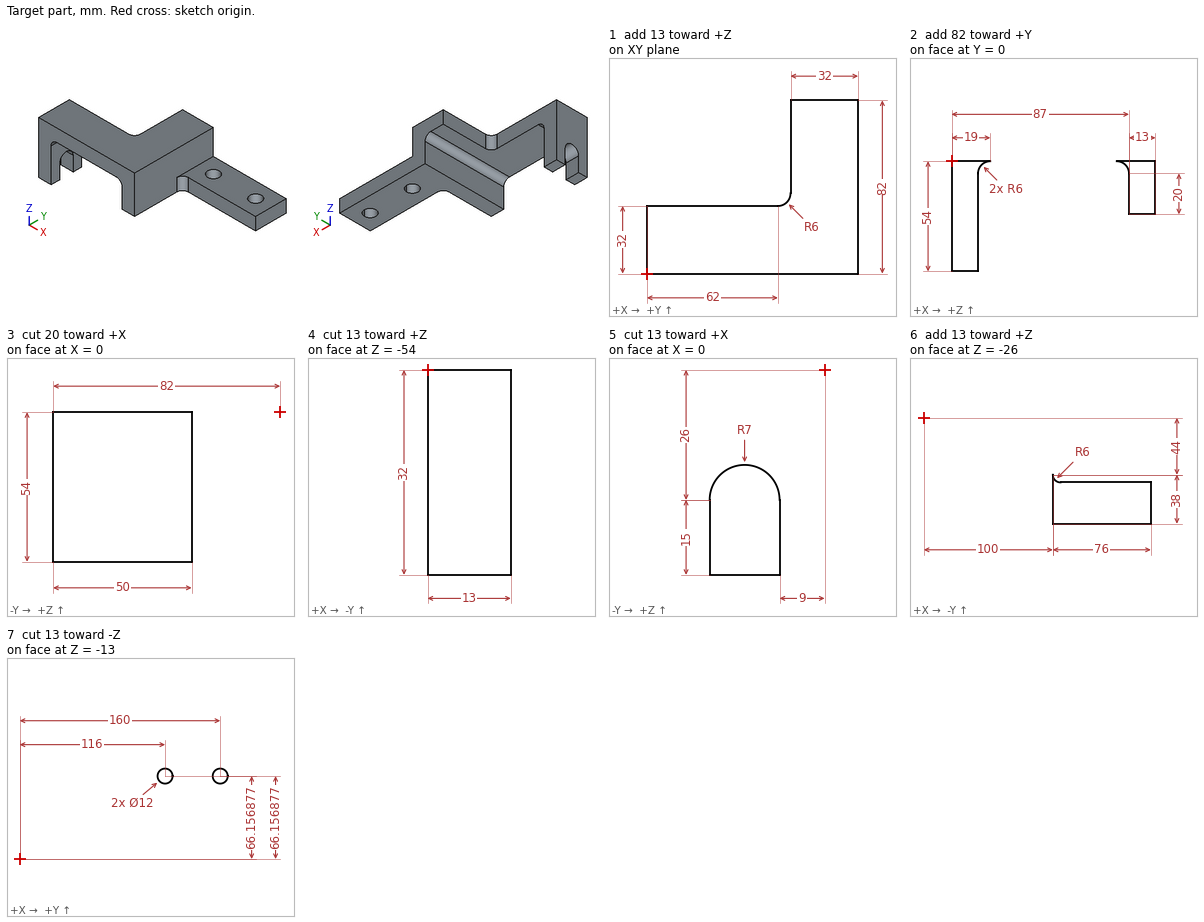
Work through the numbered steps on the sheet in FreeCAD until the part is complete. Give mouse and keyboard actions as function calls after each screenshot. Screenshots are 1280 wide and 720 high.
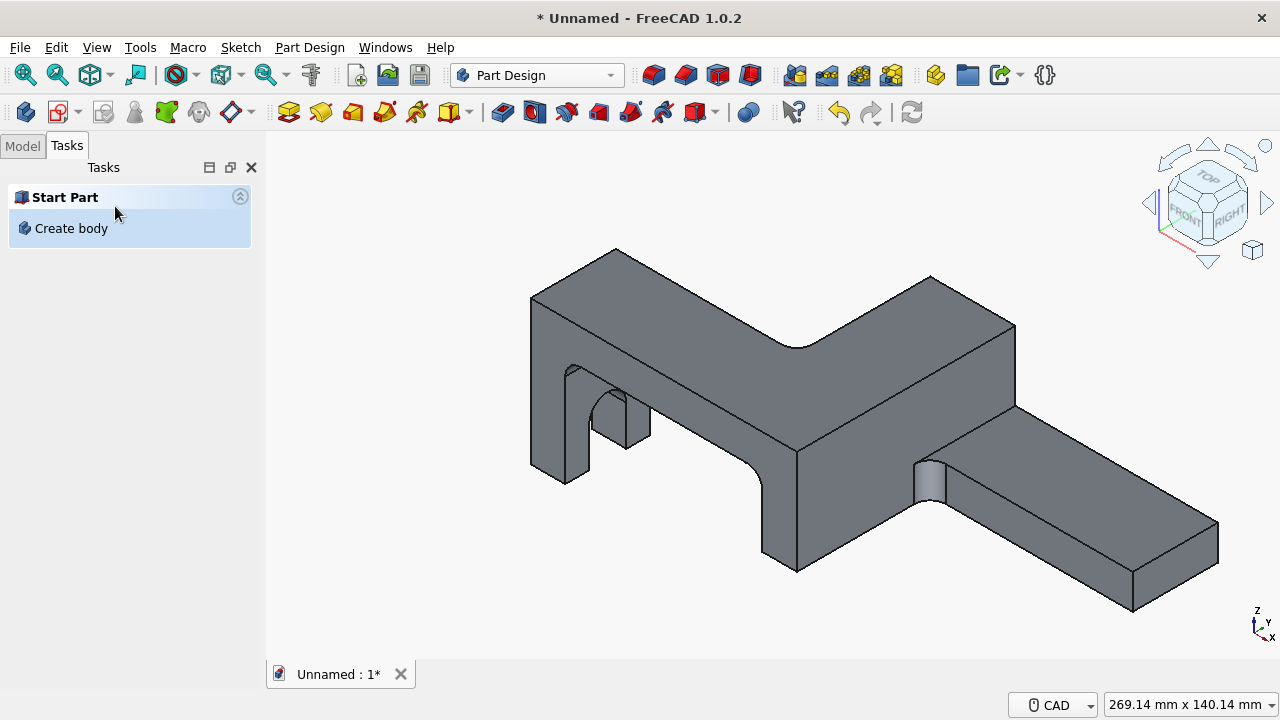
click(26, 76)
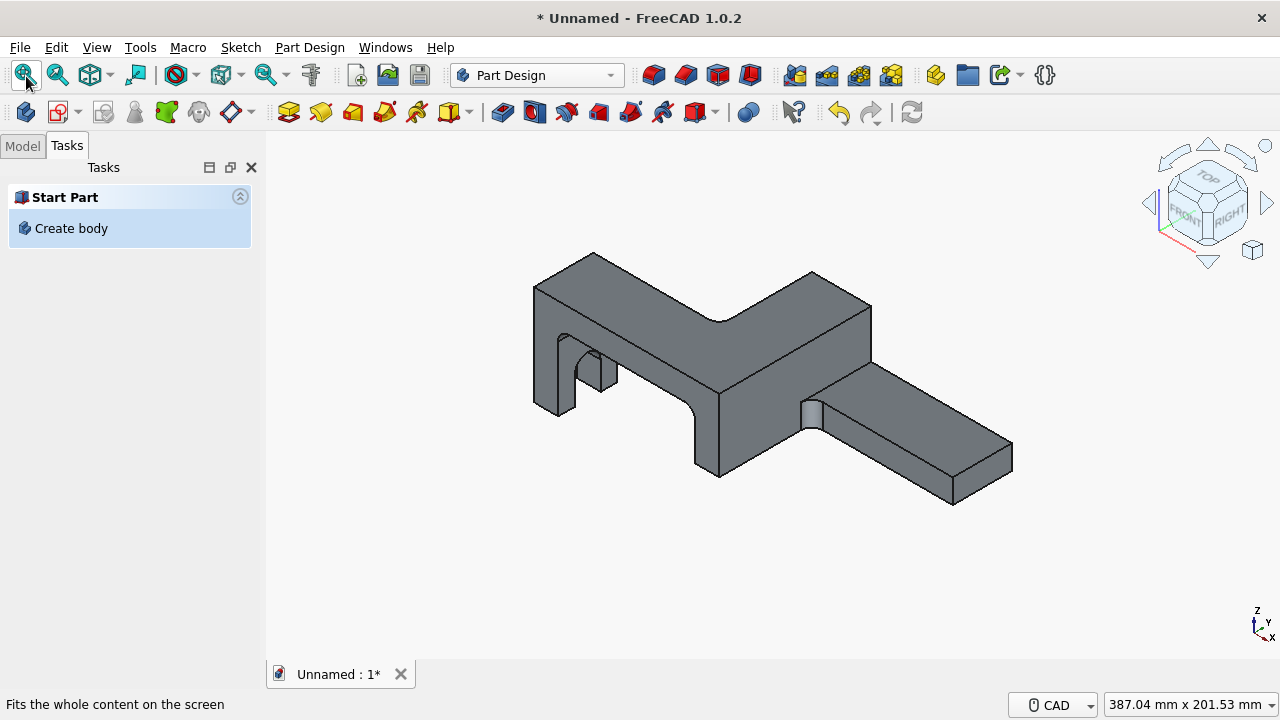
click(957, 439)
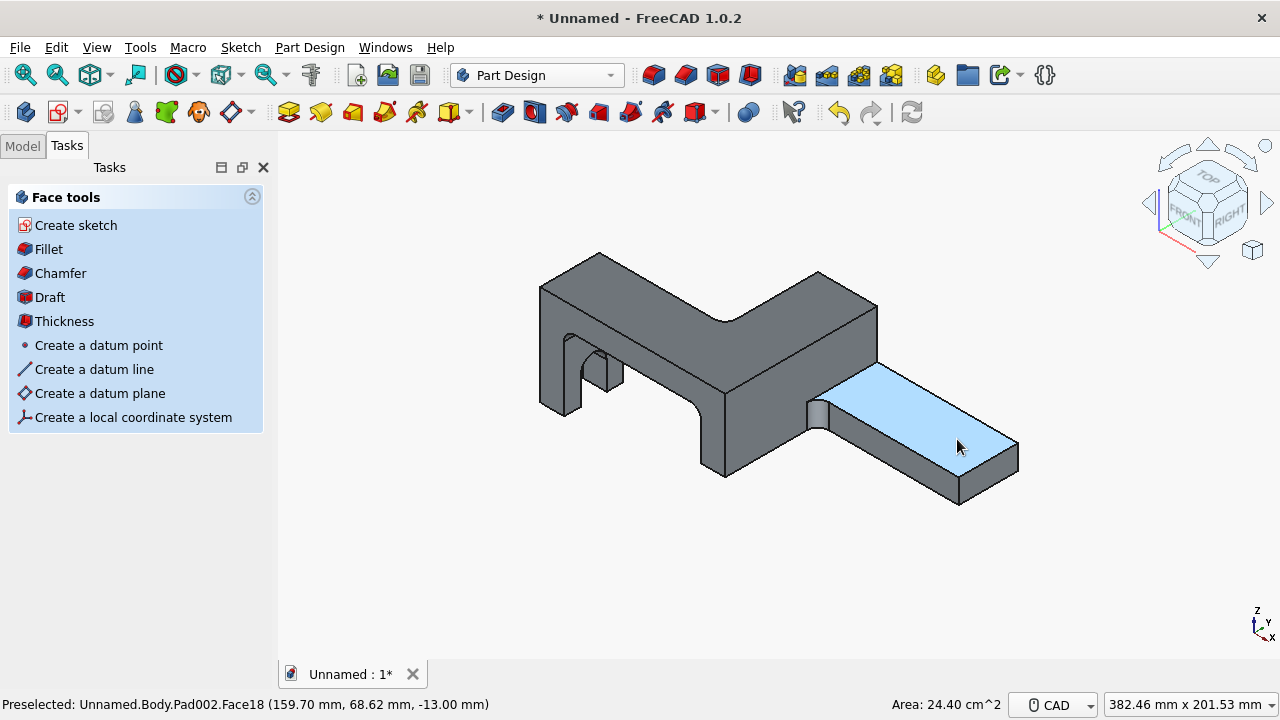
click(58, 112)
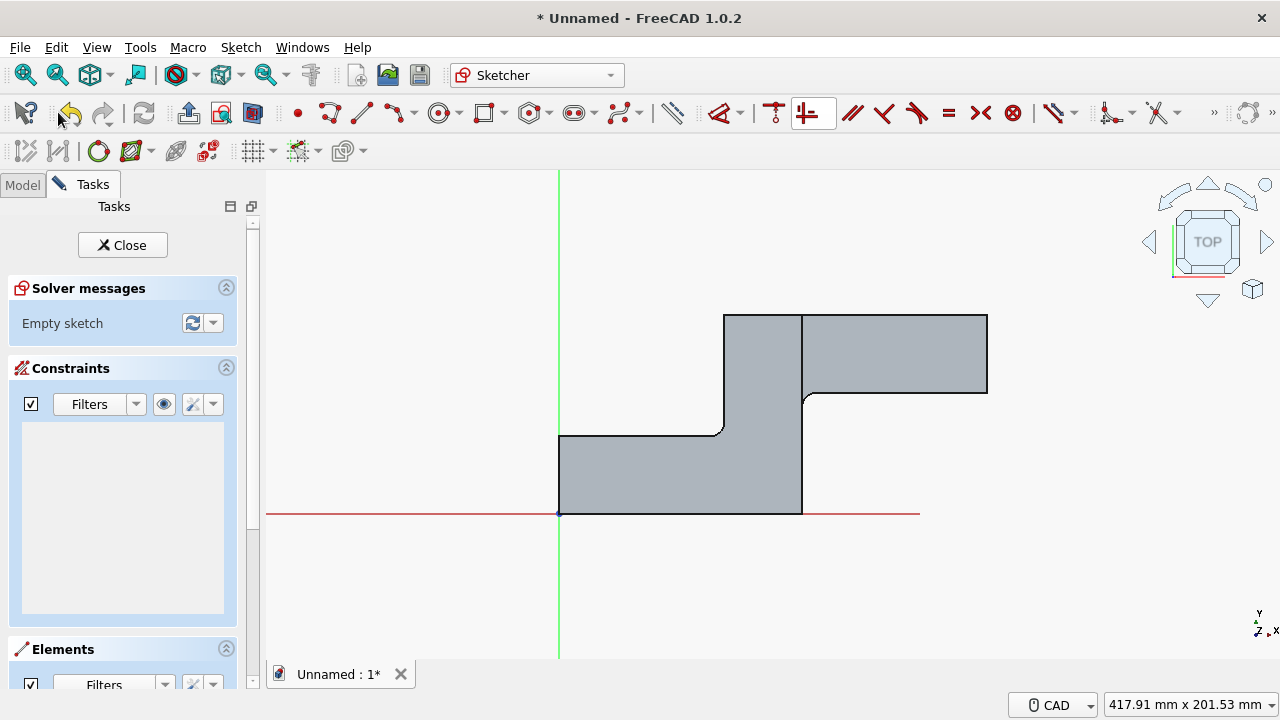
scroll(956, 333, up, 7)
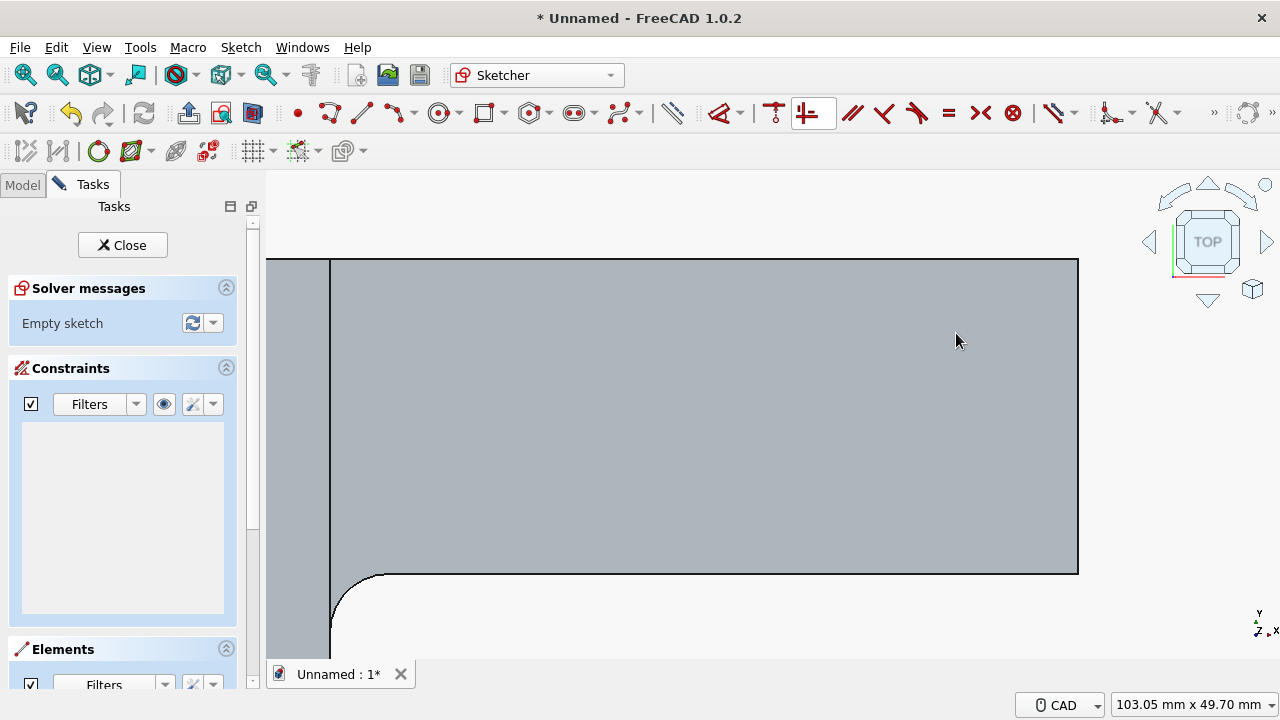
click(440, 114)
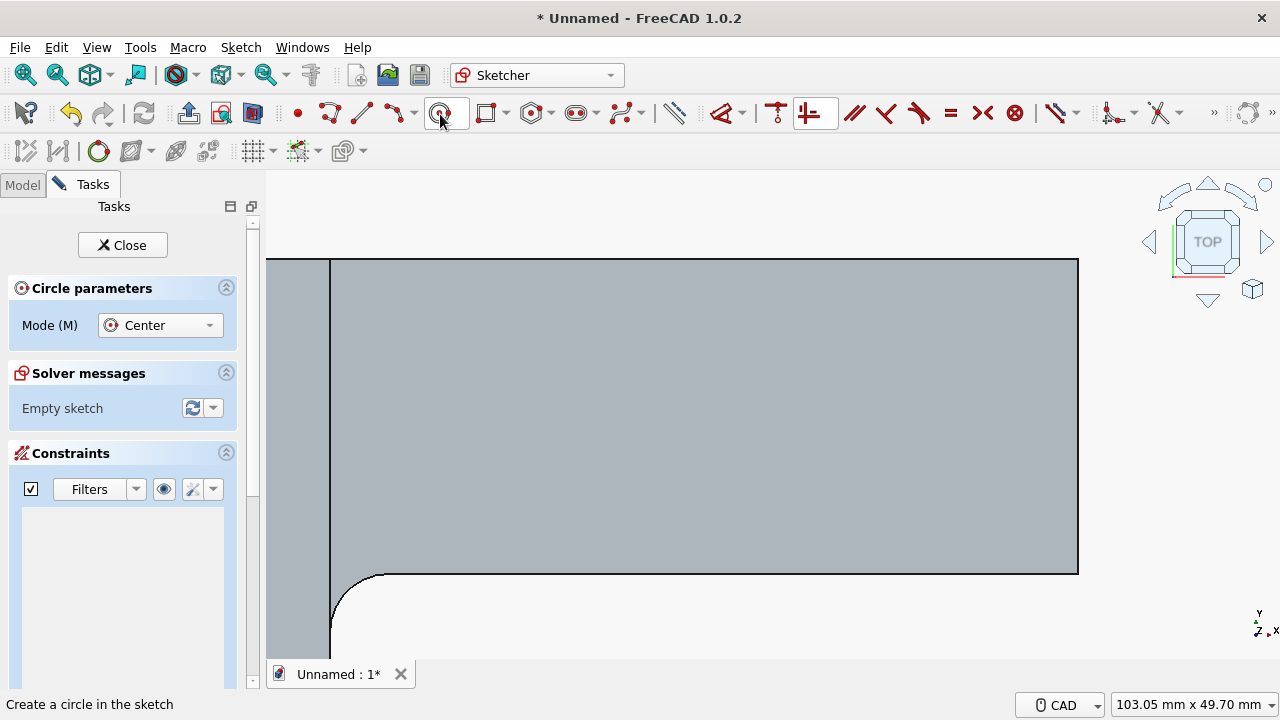
click(487, 415)
click(529, 373)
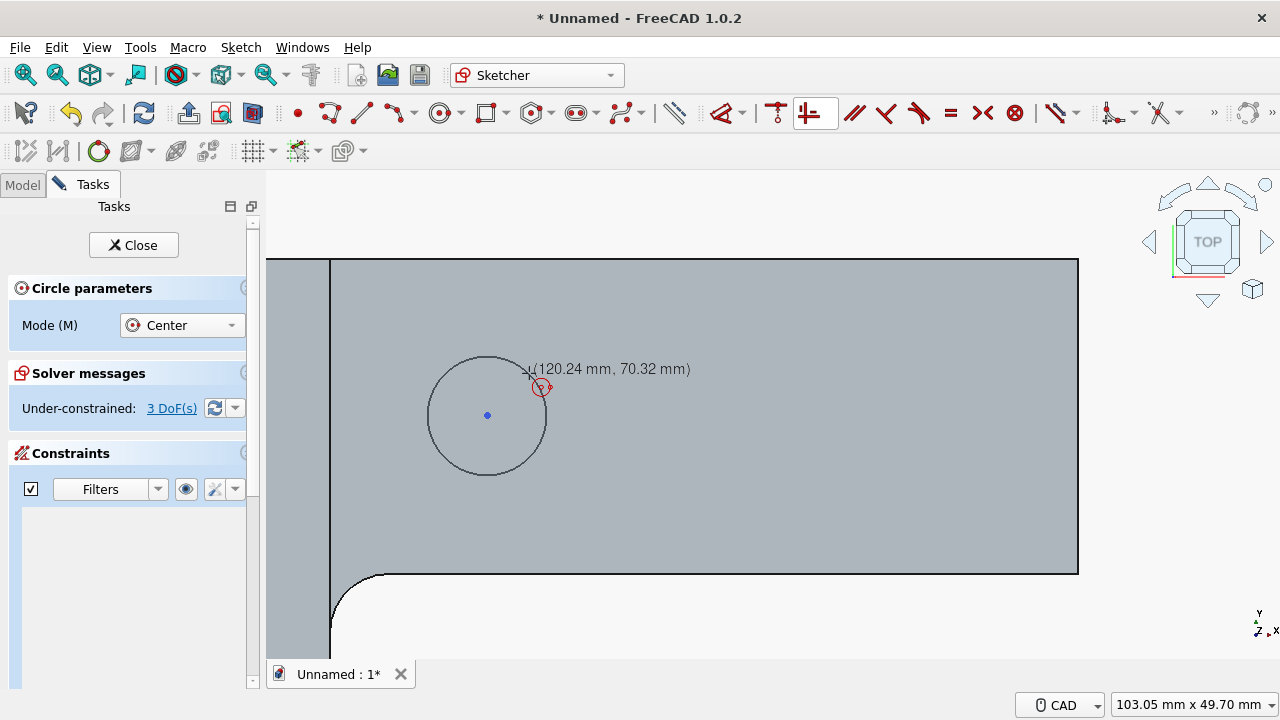
click(920, 415)
click(962, 373)
key(Escape)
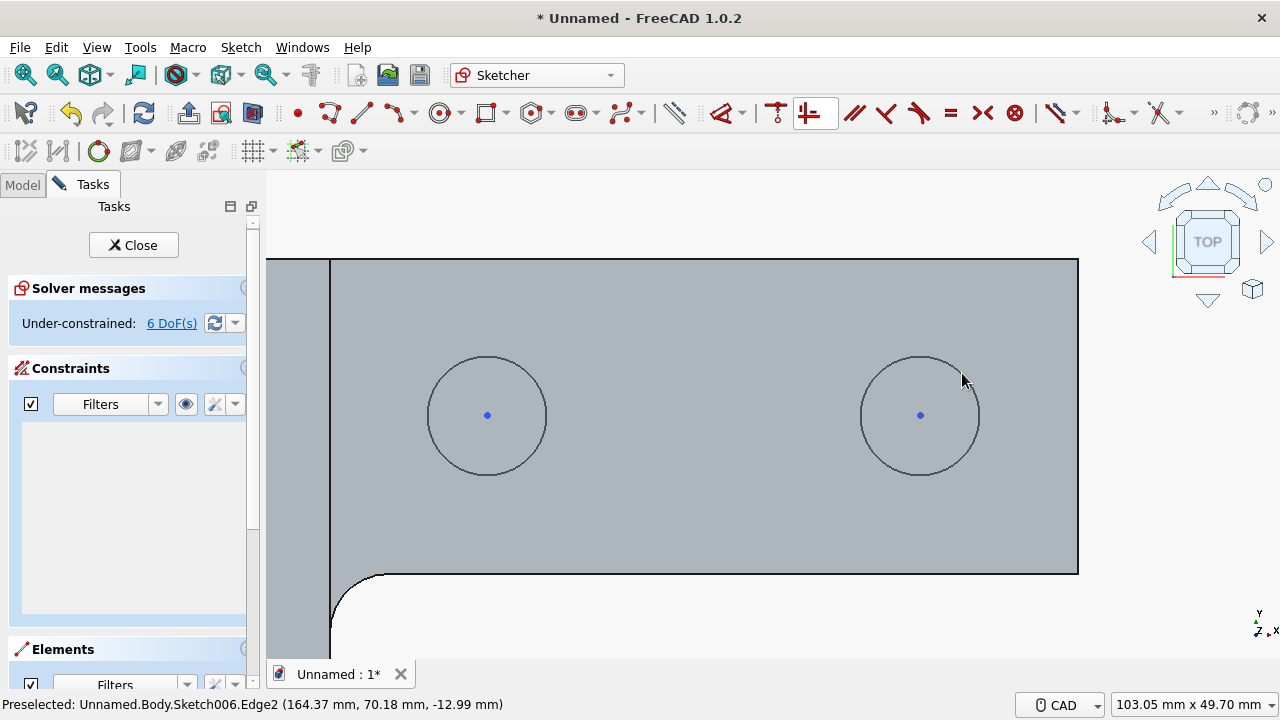
click(529, 374)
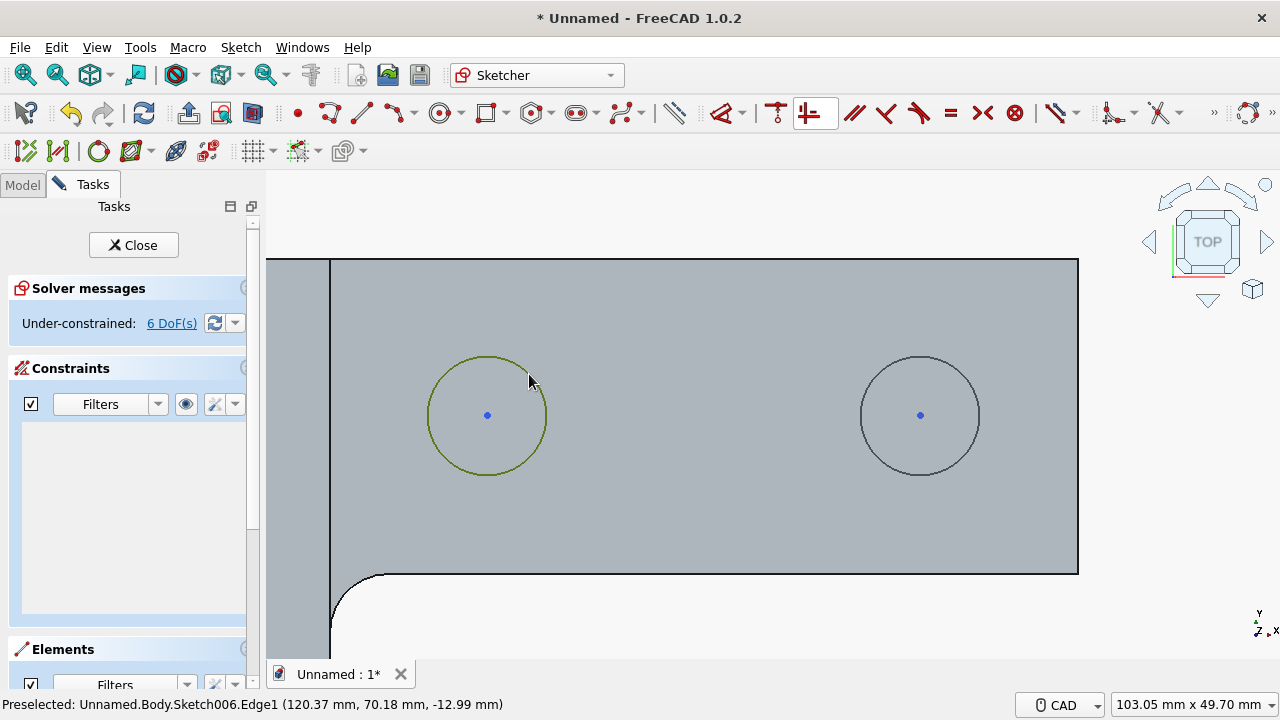
click(962, 374)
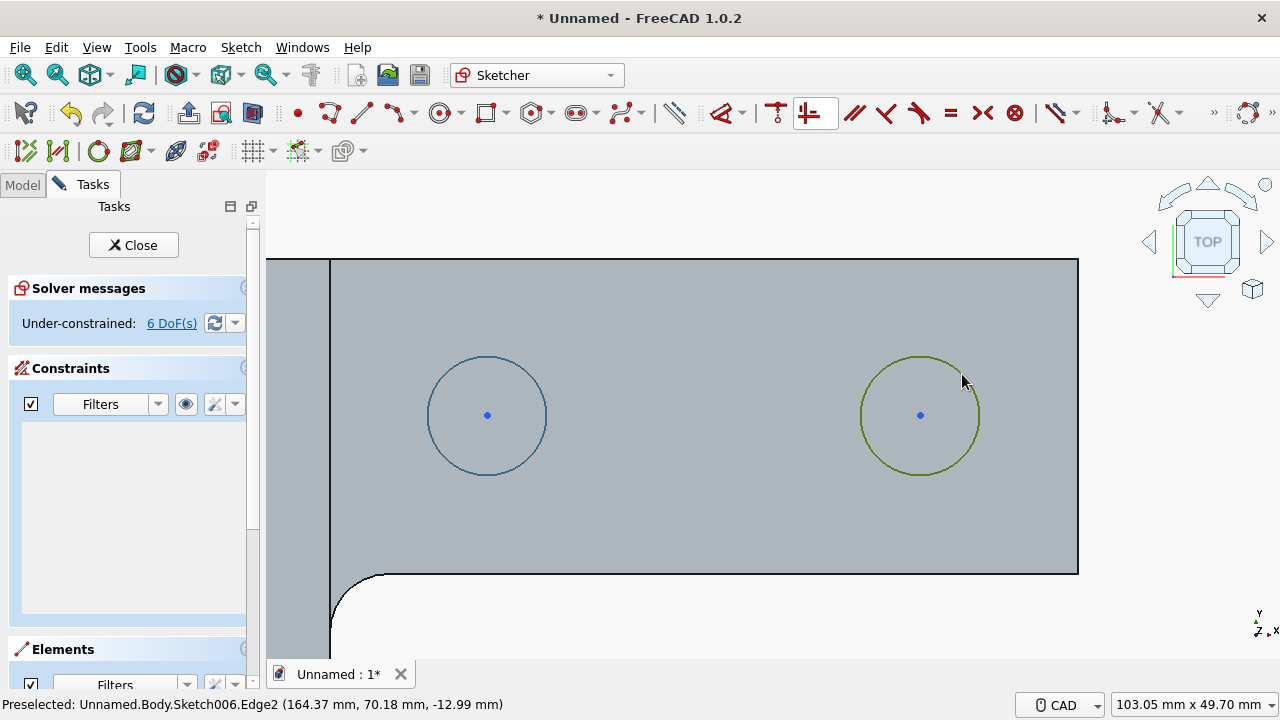
click(952, 114)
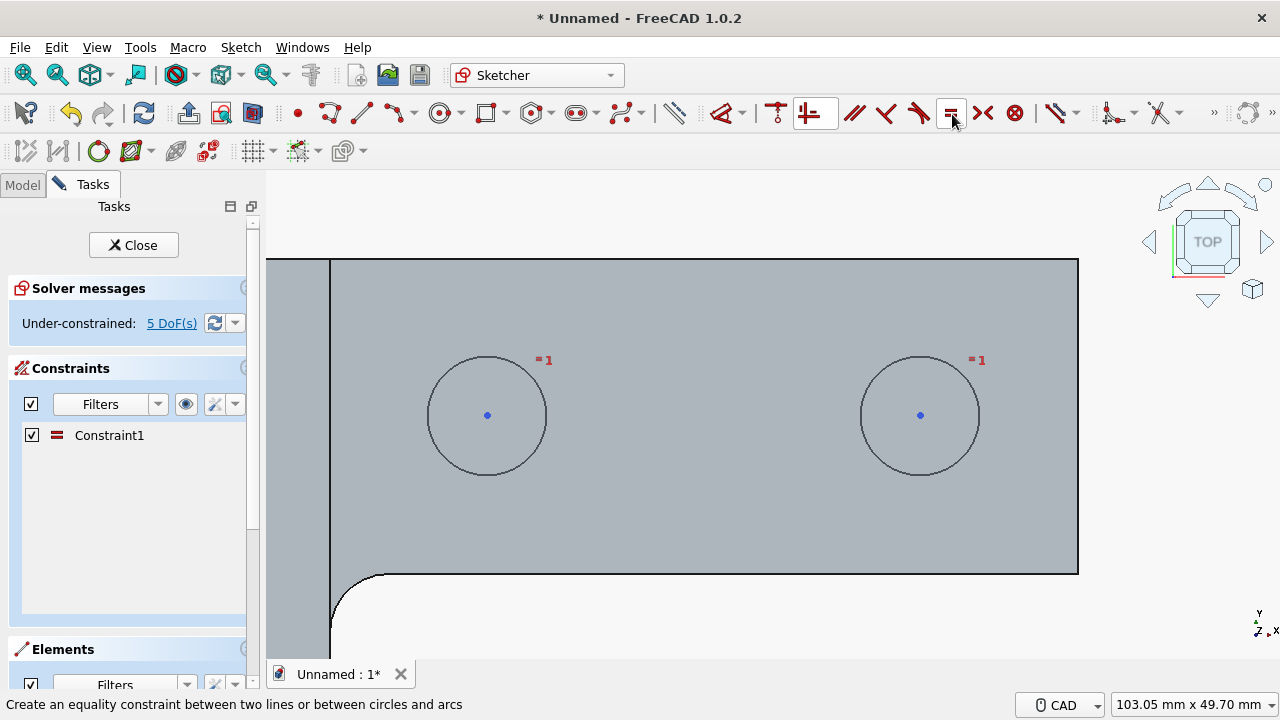
click(722, 114)